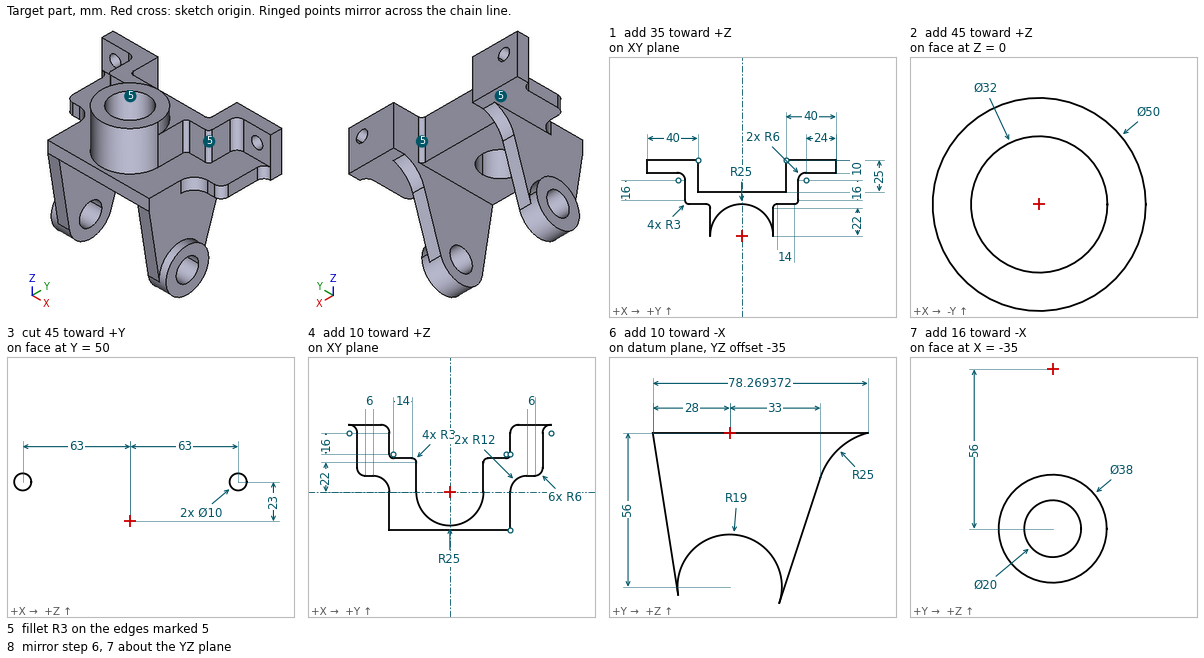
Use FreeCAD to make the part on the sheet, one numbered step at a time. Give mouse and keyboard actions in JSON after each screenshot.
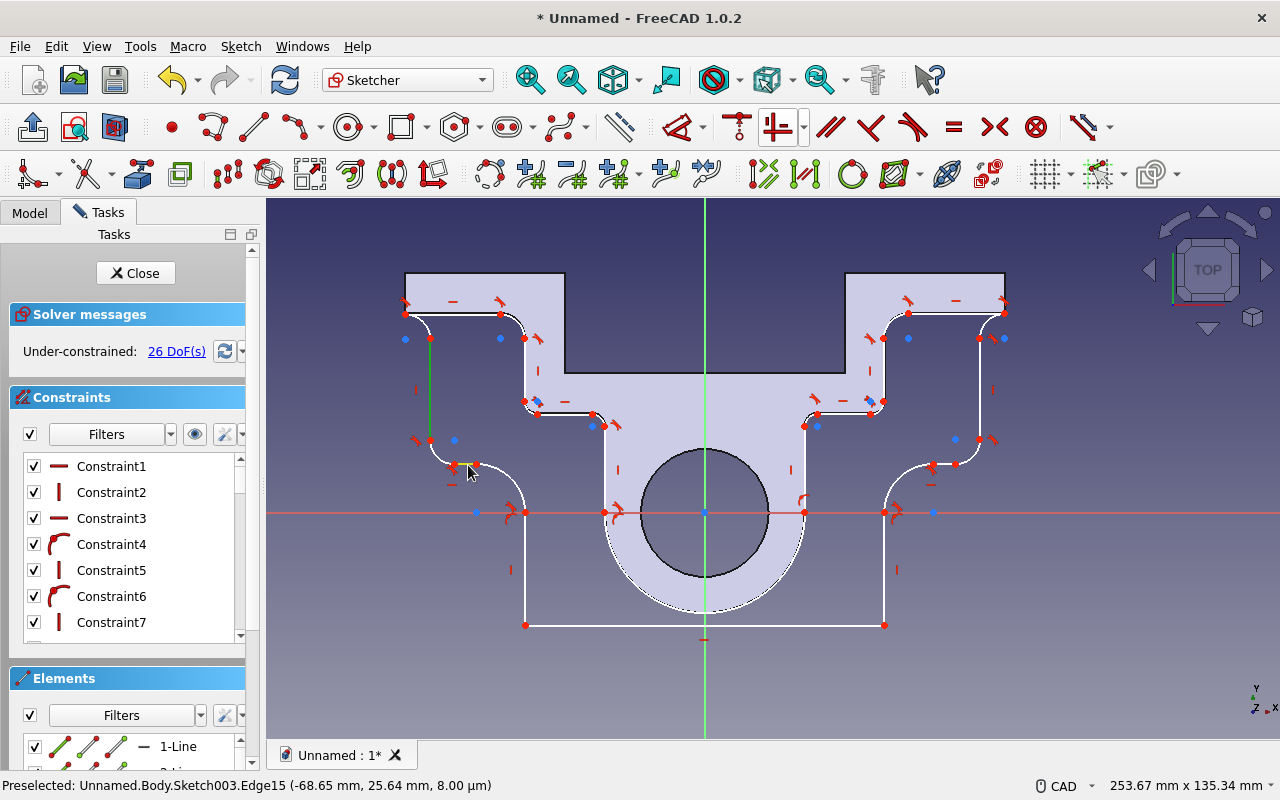
{"action": "left_click", "coordinate": [427, 328]}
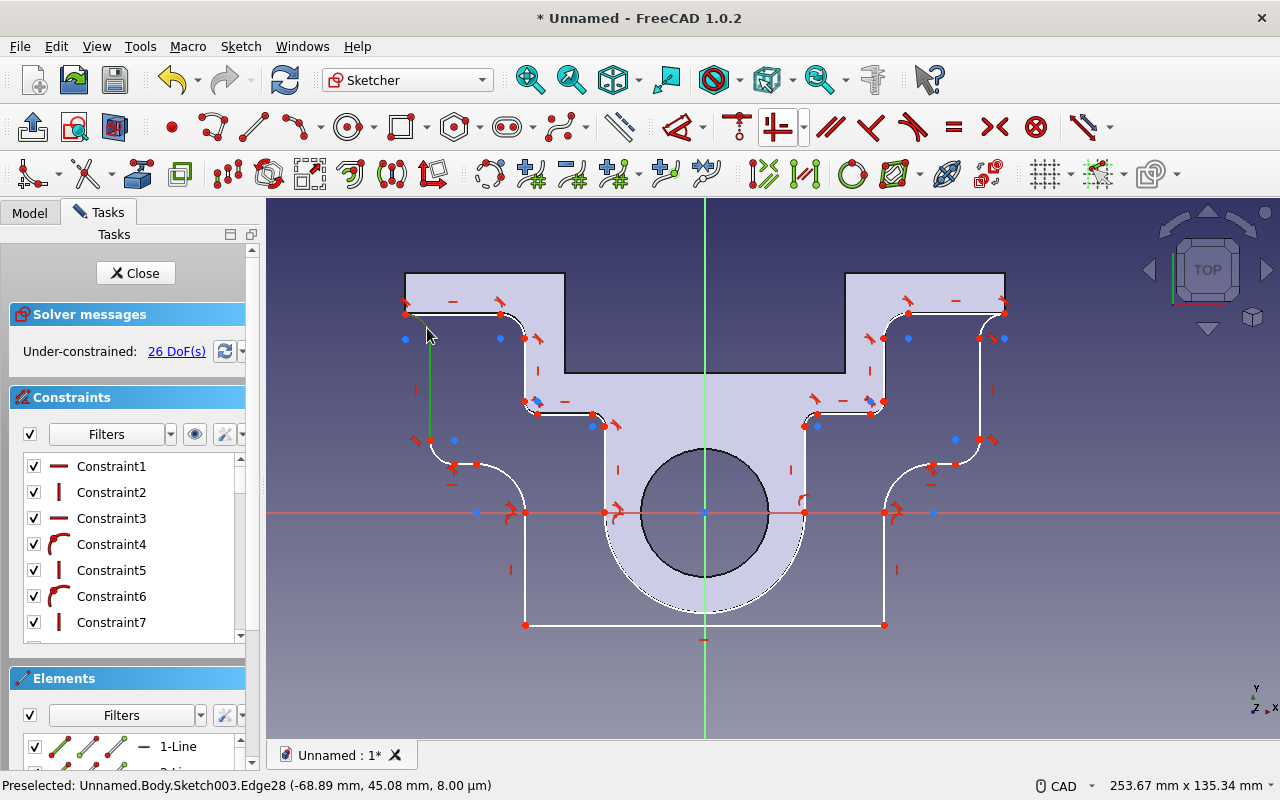
{"action": "left_click", "coordinate": [913, 128]}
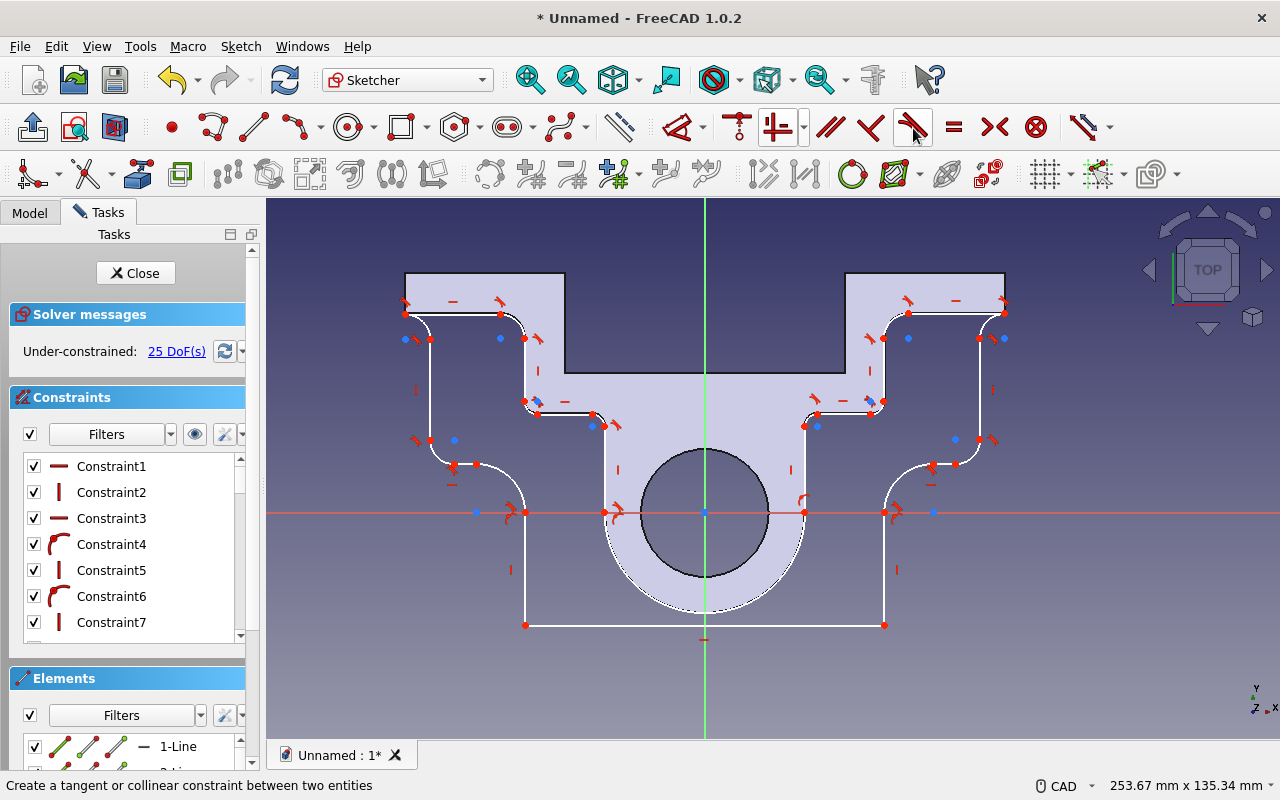
{"action": "scroll", "coordinate": [528, 411], "scroll_direction": "up", "scroll_amount": 2}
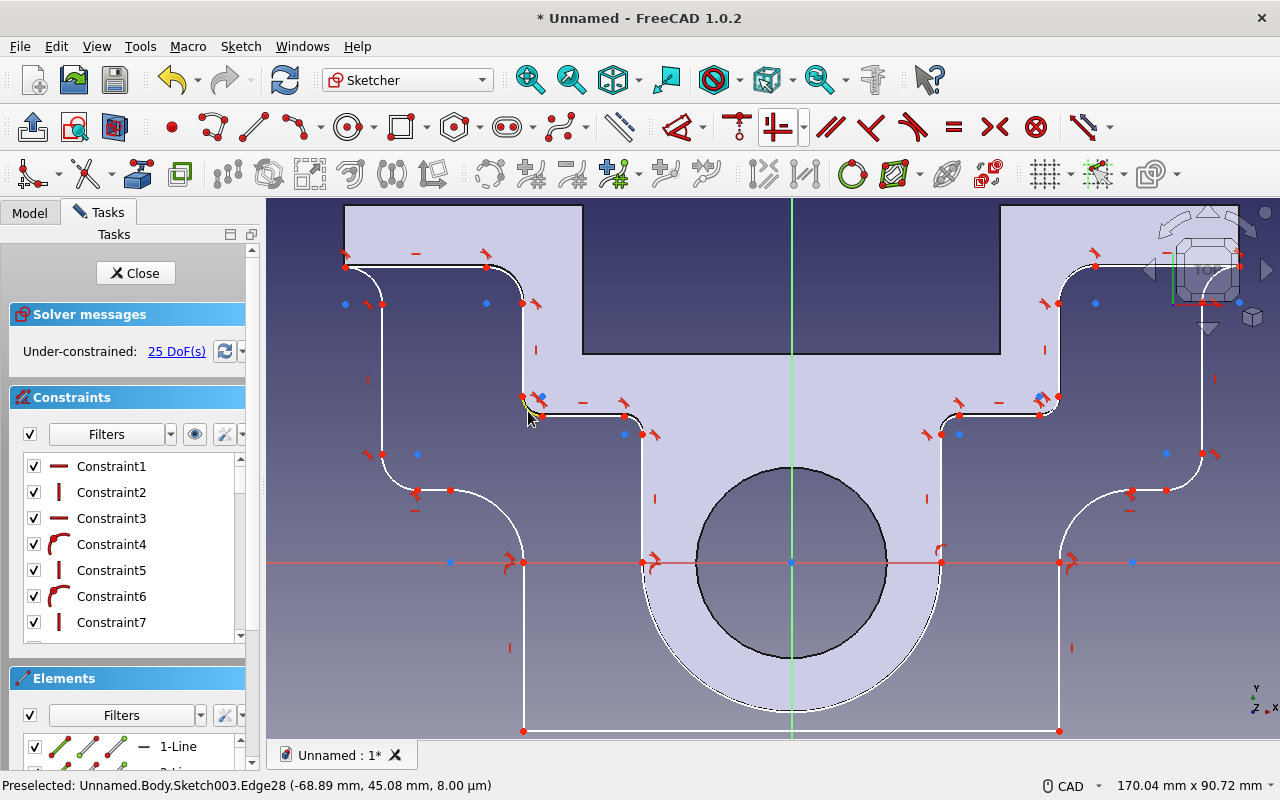
{"action": "left_click", "coordinate": [529, 410]}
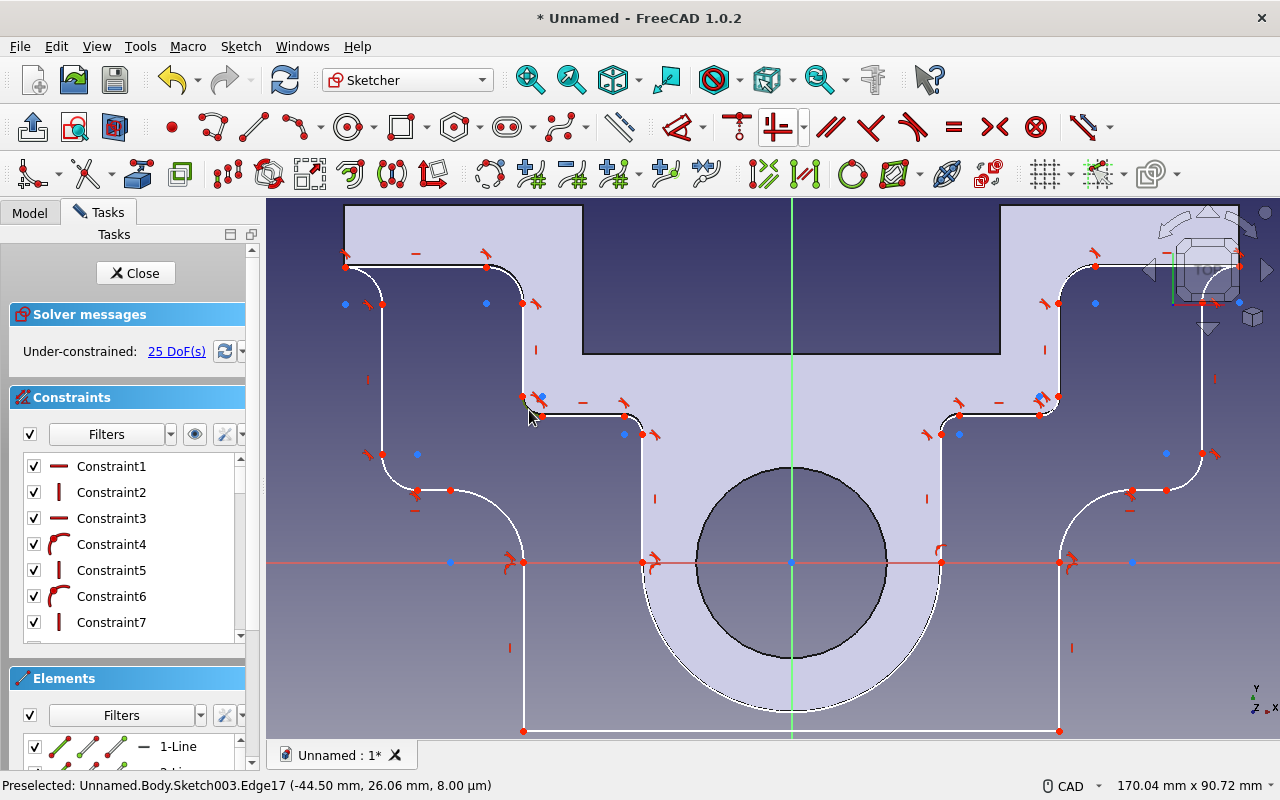
{"action": "left_click", "coordinate": [637, 421]}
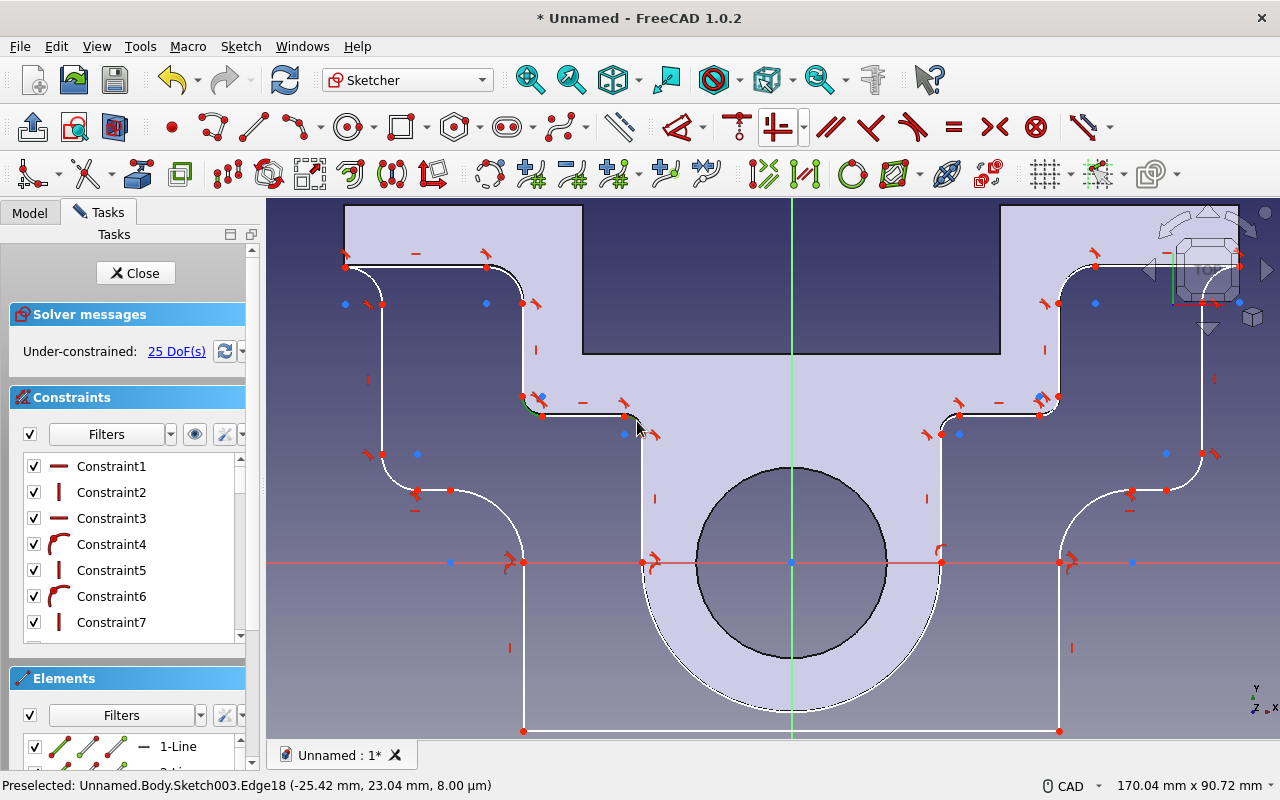
{"action": "left_click", "coordinate": [946, 421]}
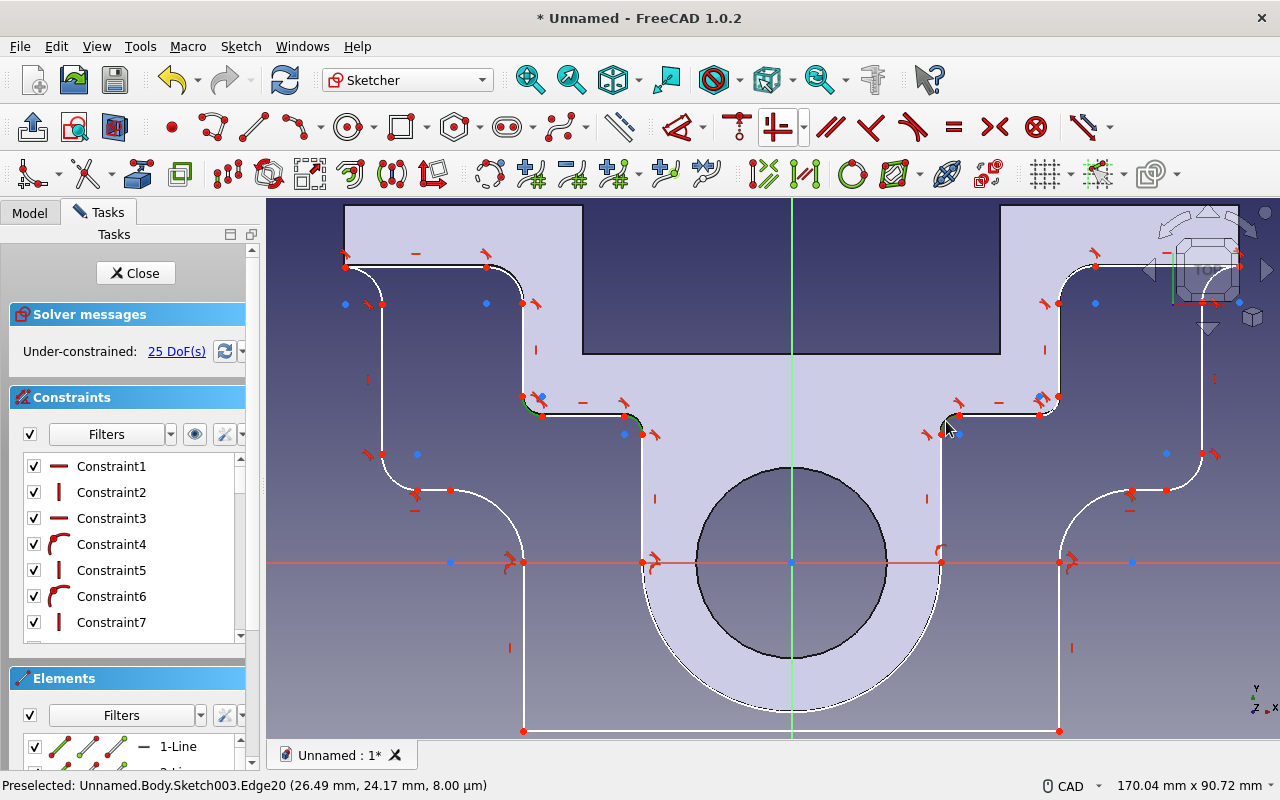
{"action": "scroll", "coordinate": [1048, 414], "scroll_direction": "up", "scroll_amount": 3}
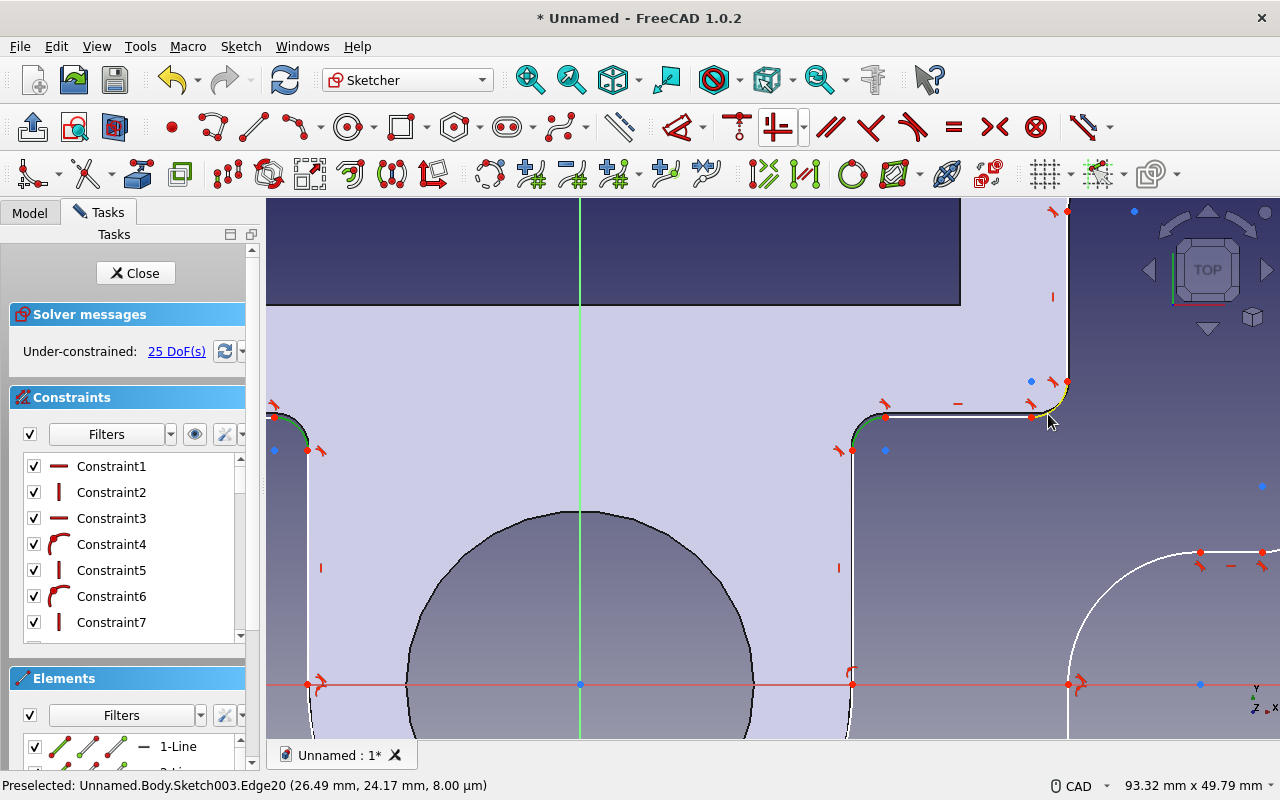
{"action": "left_click", "coordinate": [1048, 413]}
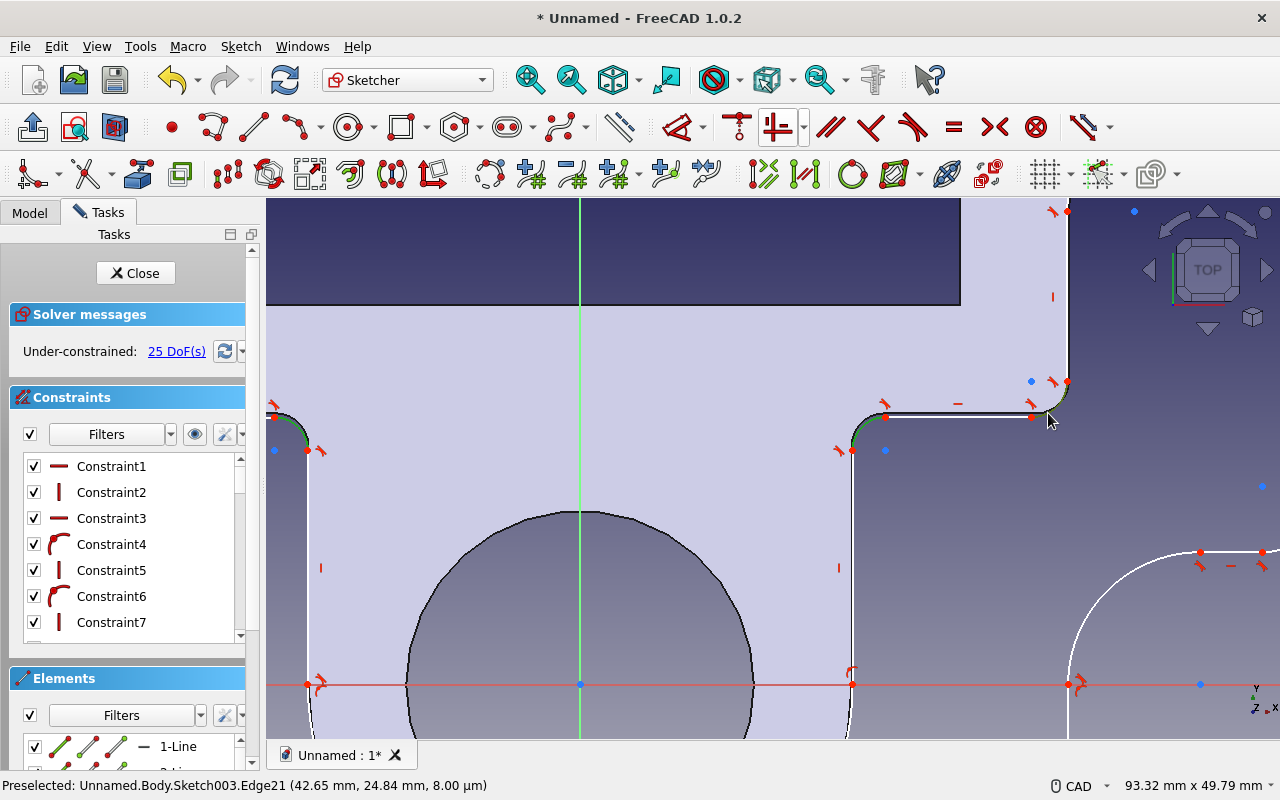
{"action": "left_click", "coordinate": [954, 128]}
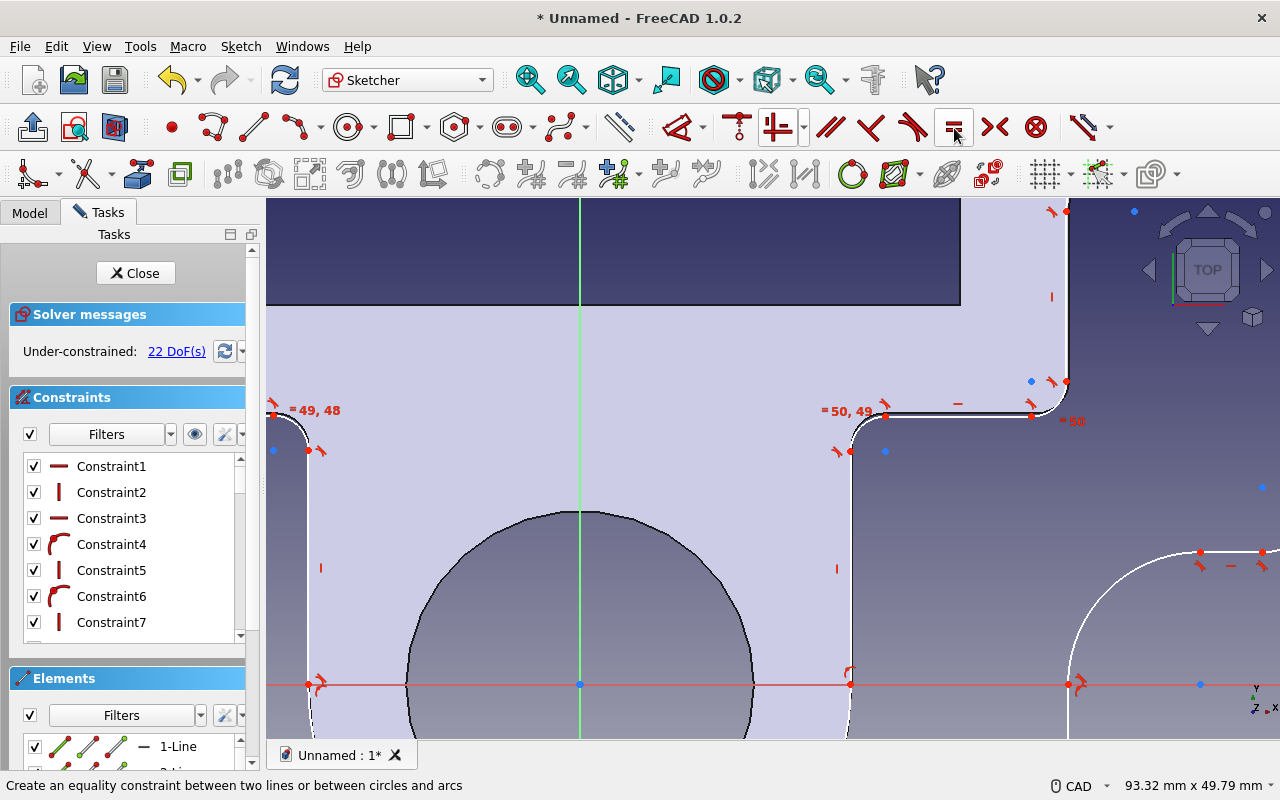
{"action": "scroll", "coordinate": [777, 412], "scroll_direction": "down", "scroll_amount": 5}